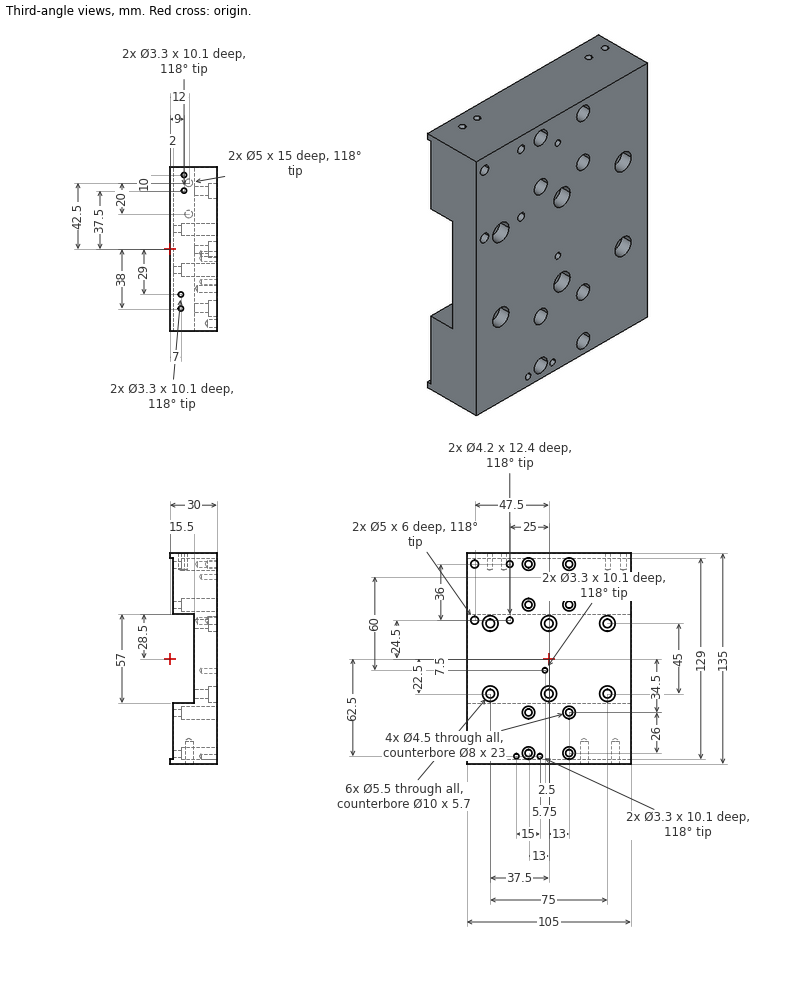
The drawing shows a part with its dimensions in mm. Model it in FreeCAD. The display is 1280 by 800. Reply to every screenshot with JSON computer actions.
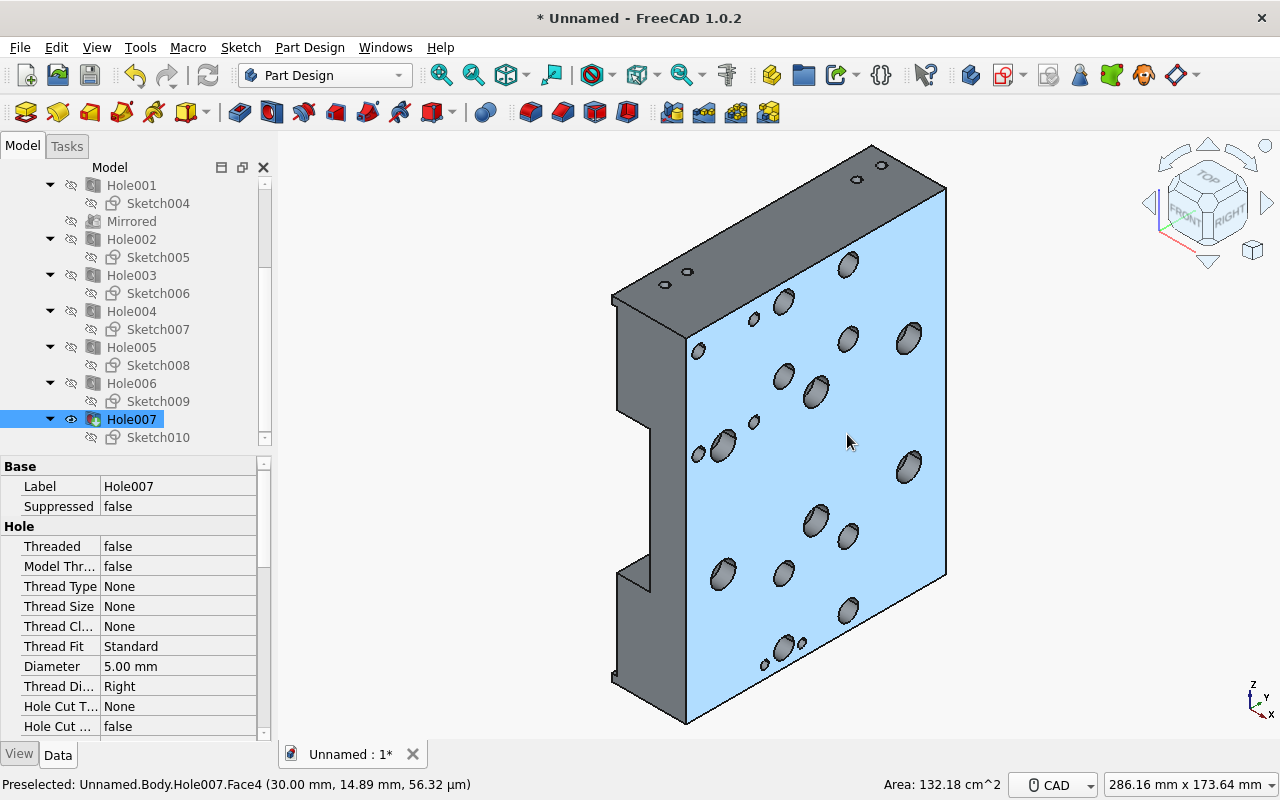
{"action": "left_click", "coordinate": [1004, 76]}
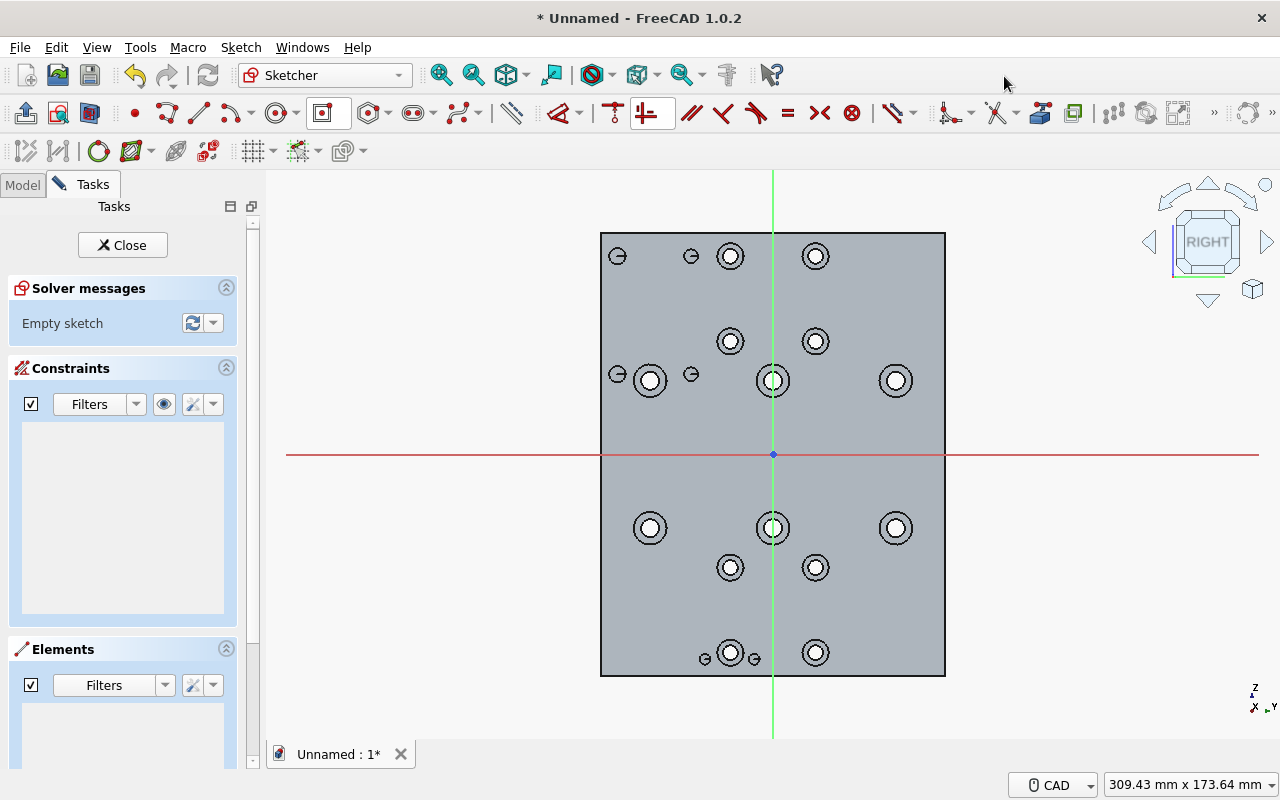
{"action": "scroll", "coordinate": [841, 291], "scroll_direction": "up", "scroll_amount": 3}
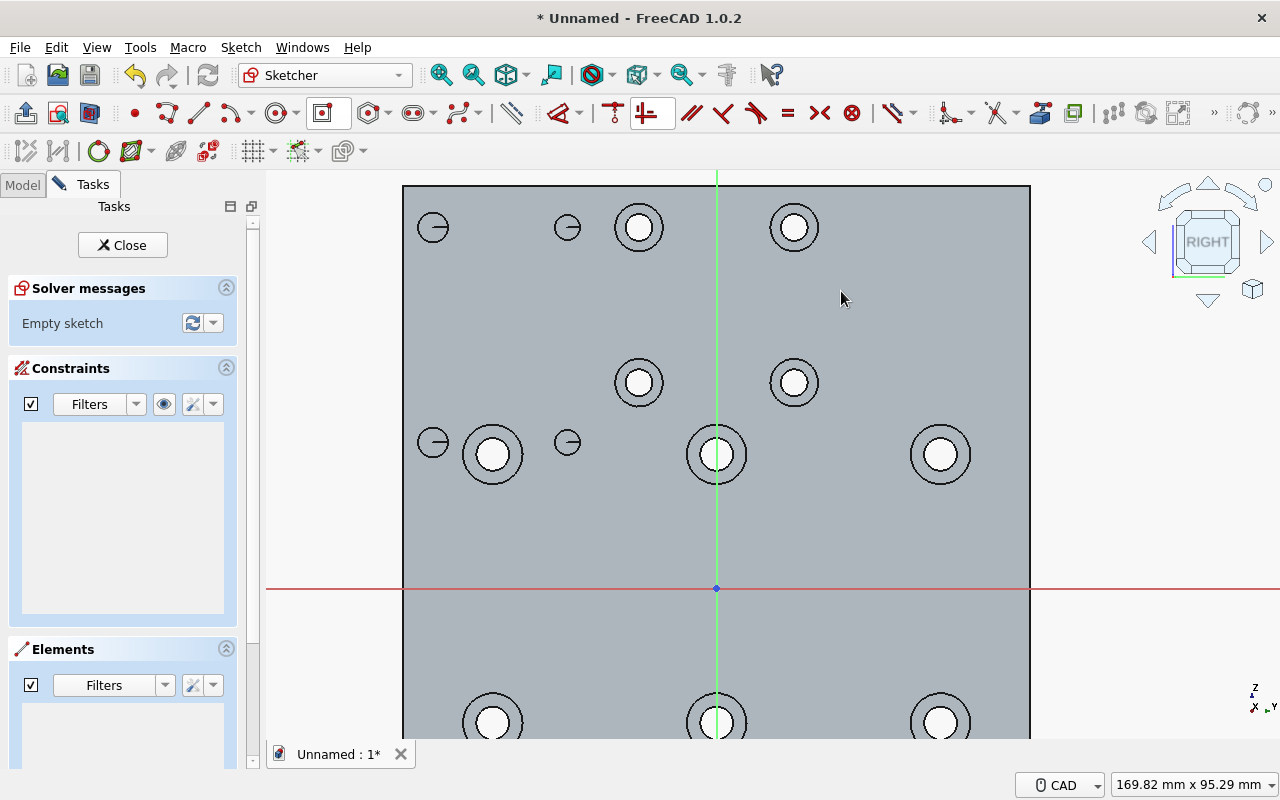
{"action": "left_click", "coordinate": [276, 114]}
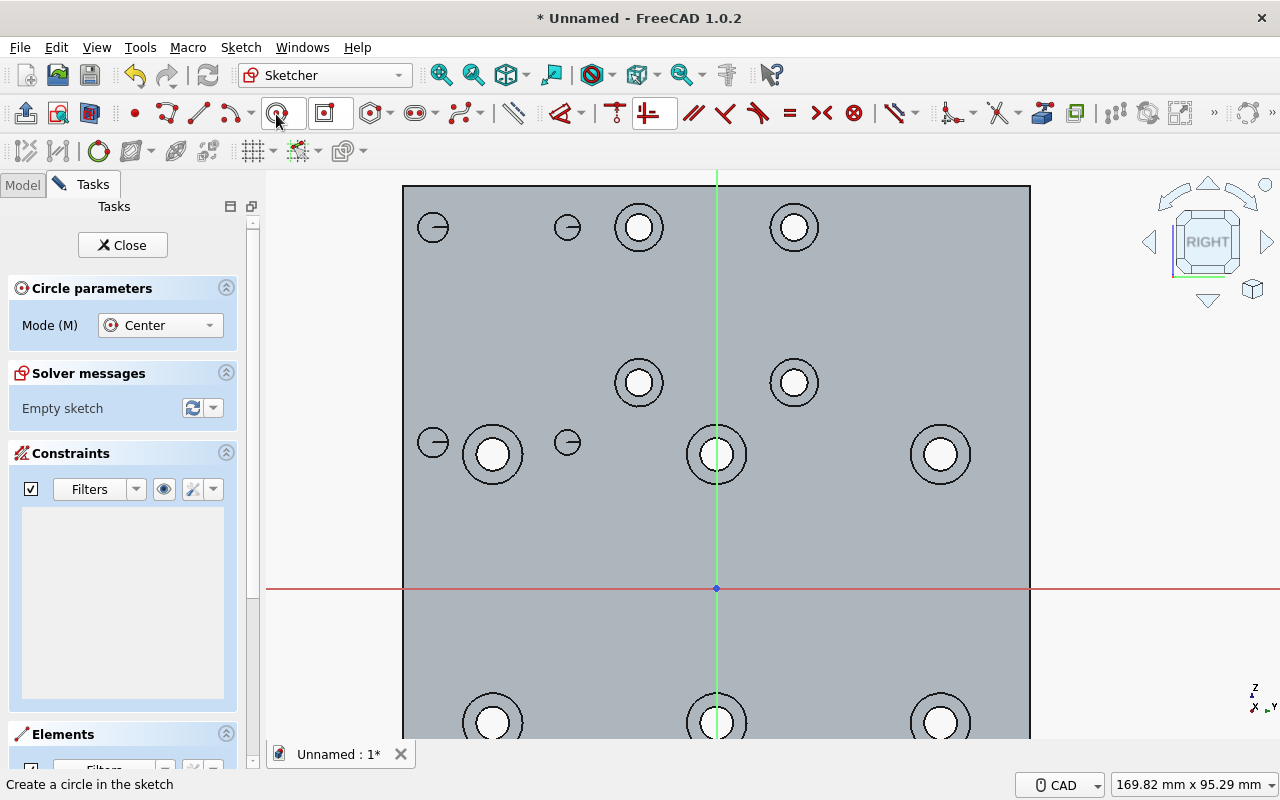
{"action": "scroll", "coordinate": [702, 634], "scroll_direction": "up", "scroll_amount": 5}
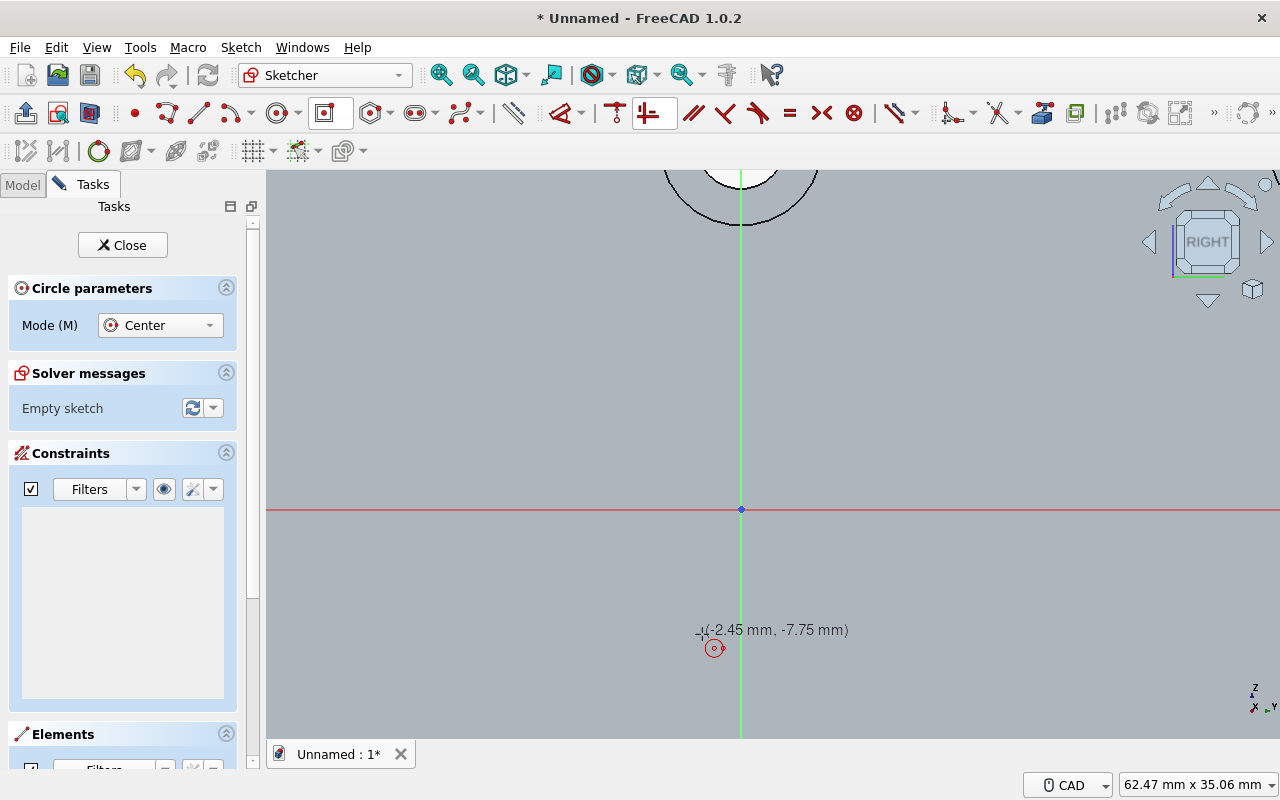
{"action": "left_click", "coordinate": [700, 631]}
{"action": "left_click", "coordinate": [719, 612]}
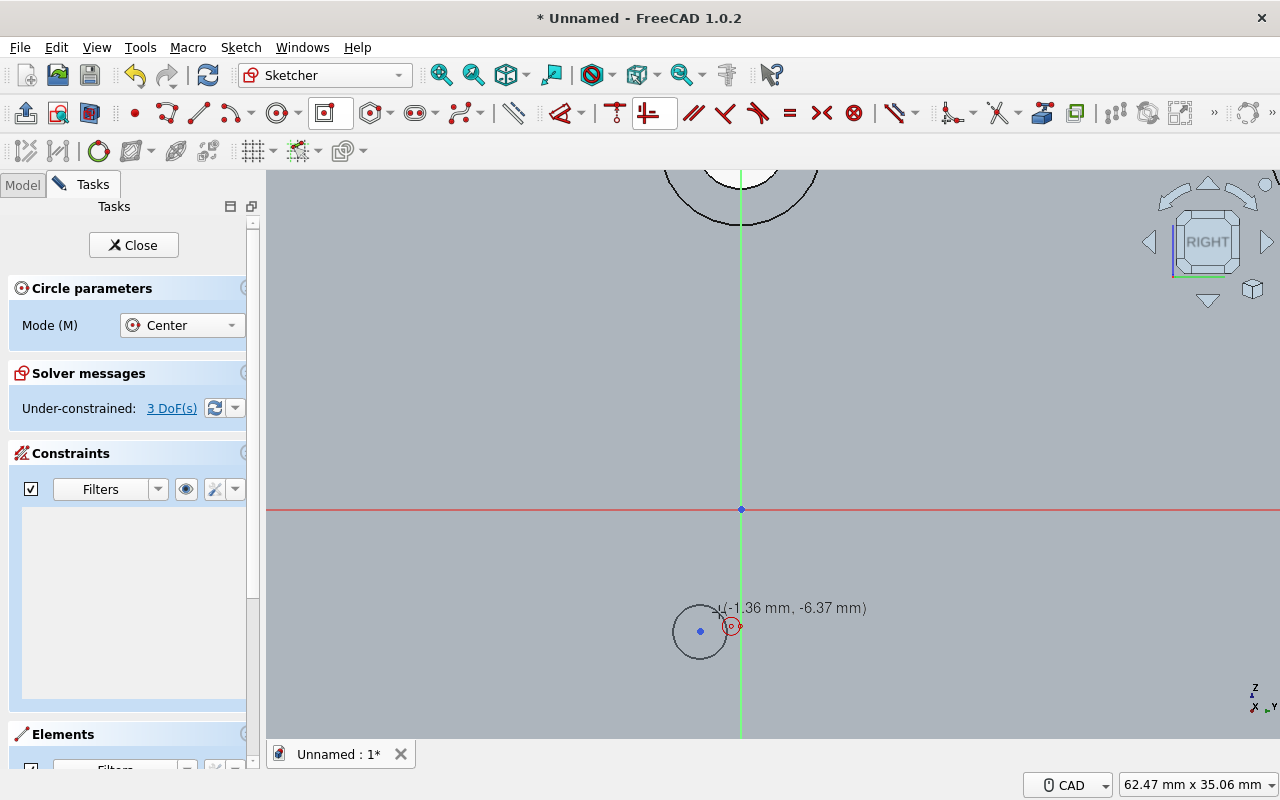
{"action": "scroll", "coordinate": [703, 635], "scroll_direction": "down", "scroll_amount": 5}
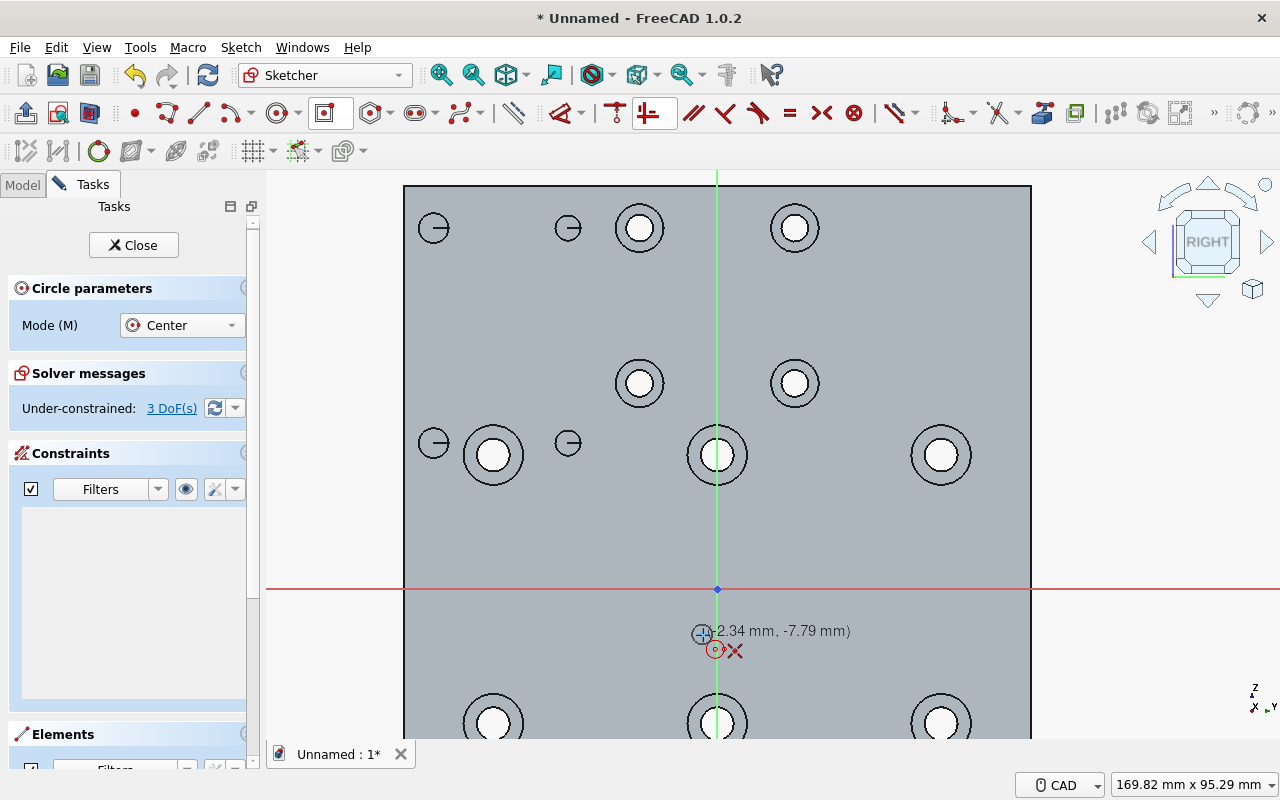
{"action": "scroll", "coordinate": [702, 276], "scroll_direction": "up", "scroll_amount": 5}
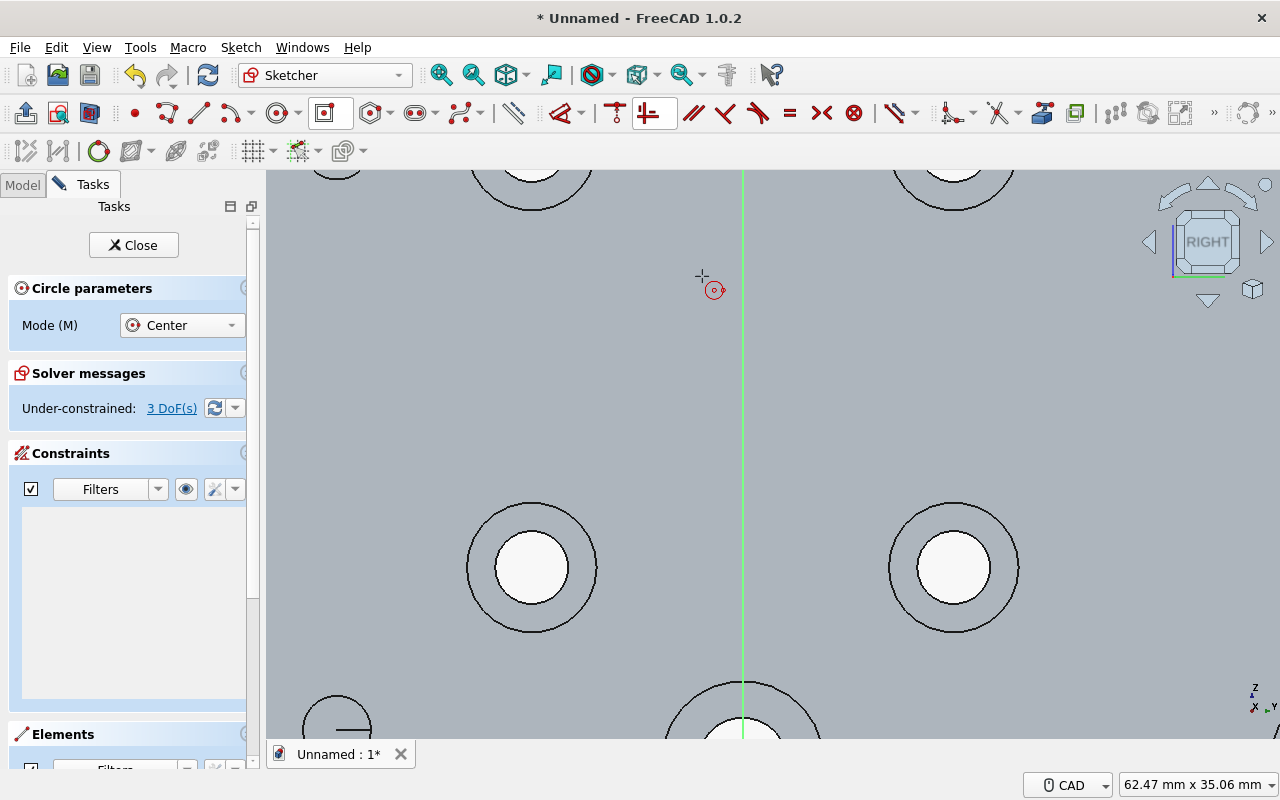
{"action": "left_click", "coordinate": [702, 275]}
{"action": "left_click", "coordinate": [721, 256]}
{"action": "key", "text": "Escape"}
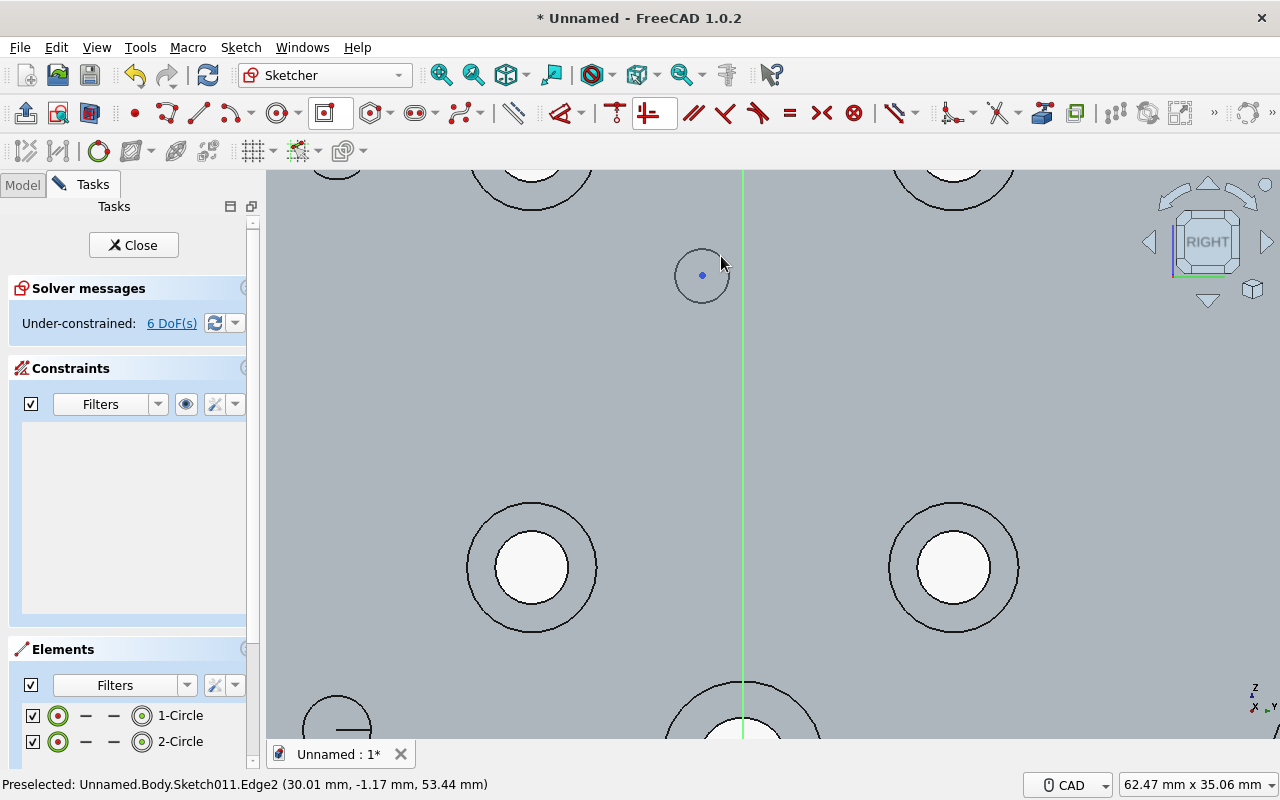
{"action": "scroll", "coordinate": [702, 275], "scroll_direction": "down", "scroll_amount": 5}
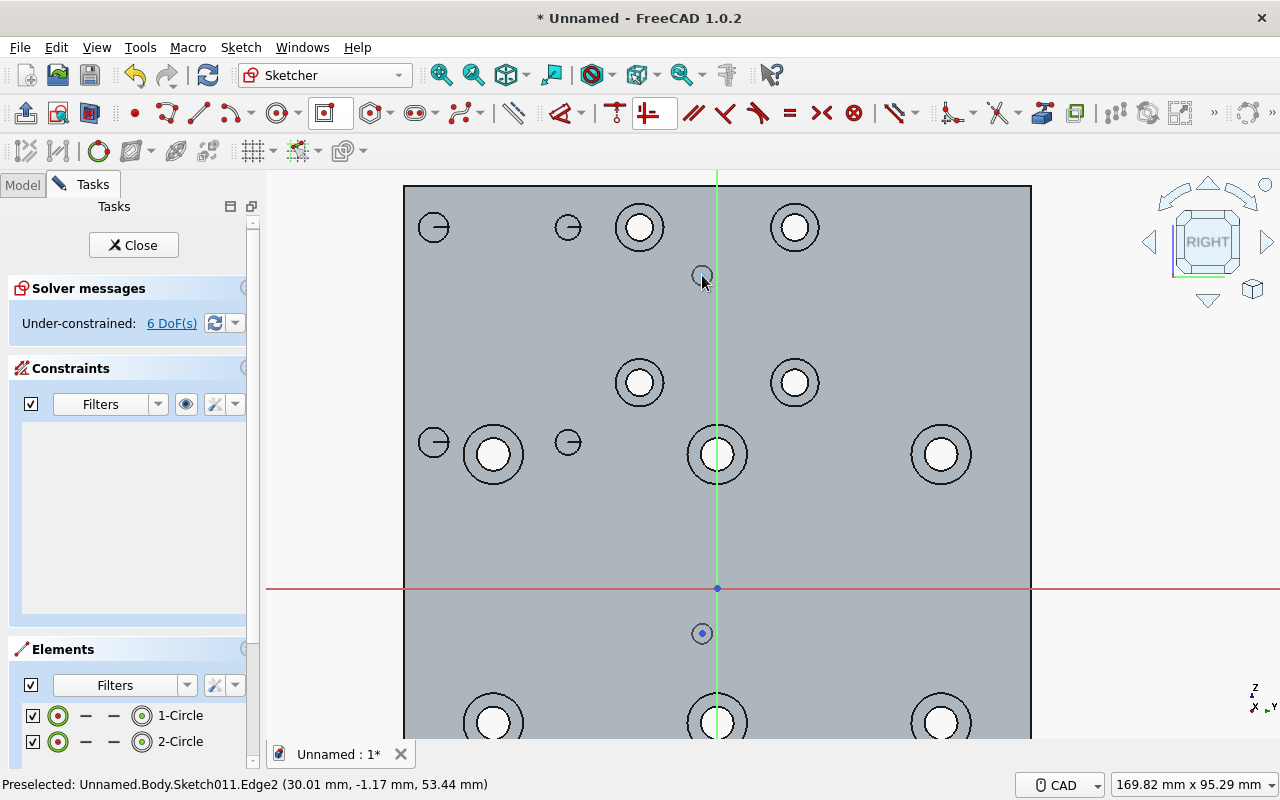
{"action": "scroll", "coordinate": [709, 627], "scroll_direction": "up", "scroll_amount": 3}